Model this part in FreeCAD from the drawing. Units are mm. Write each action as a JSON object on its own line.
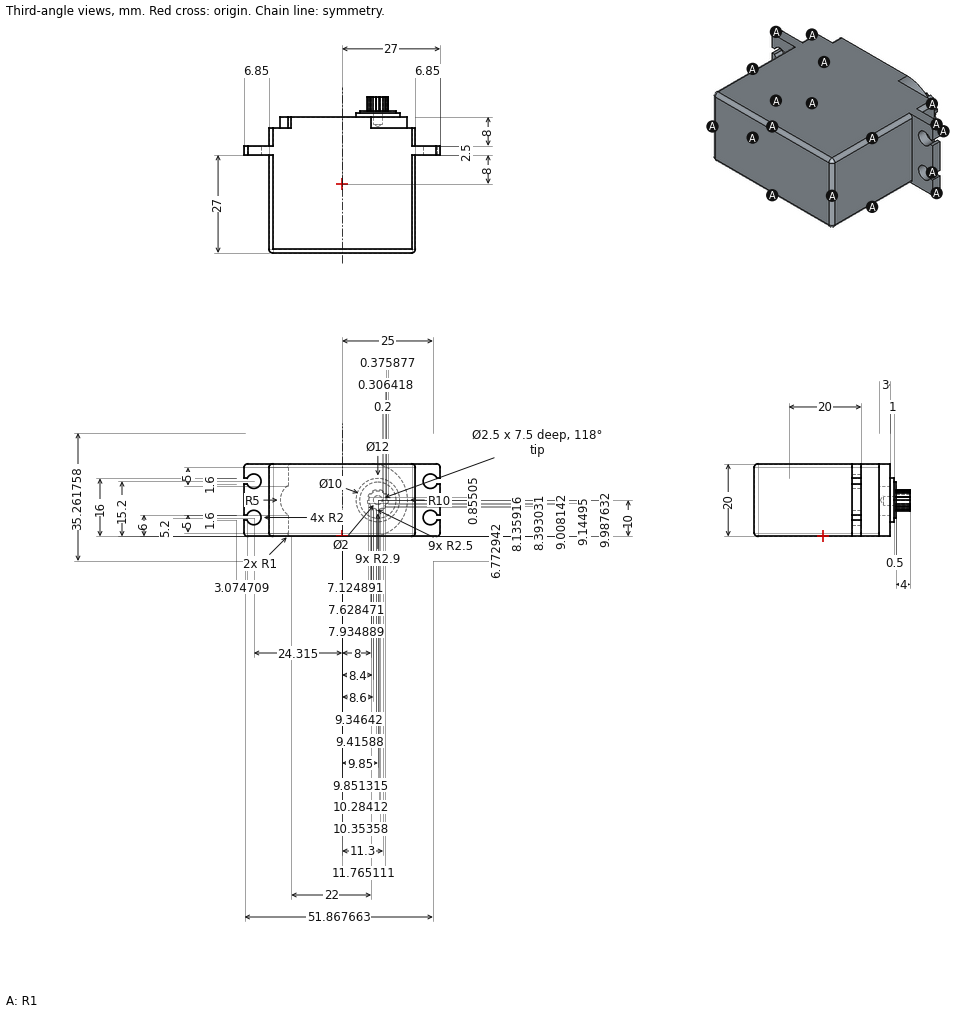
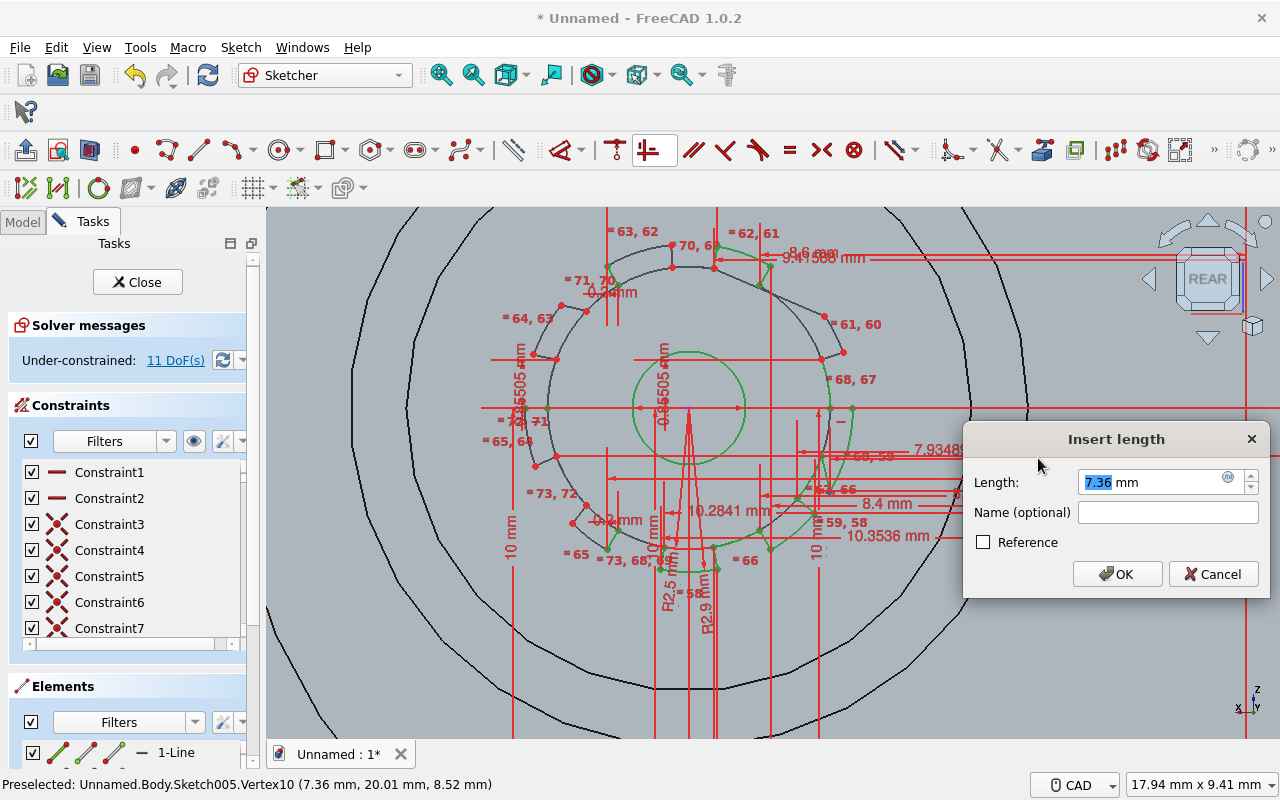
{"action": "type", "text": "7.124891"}
{"action": "key", "text": "Return"}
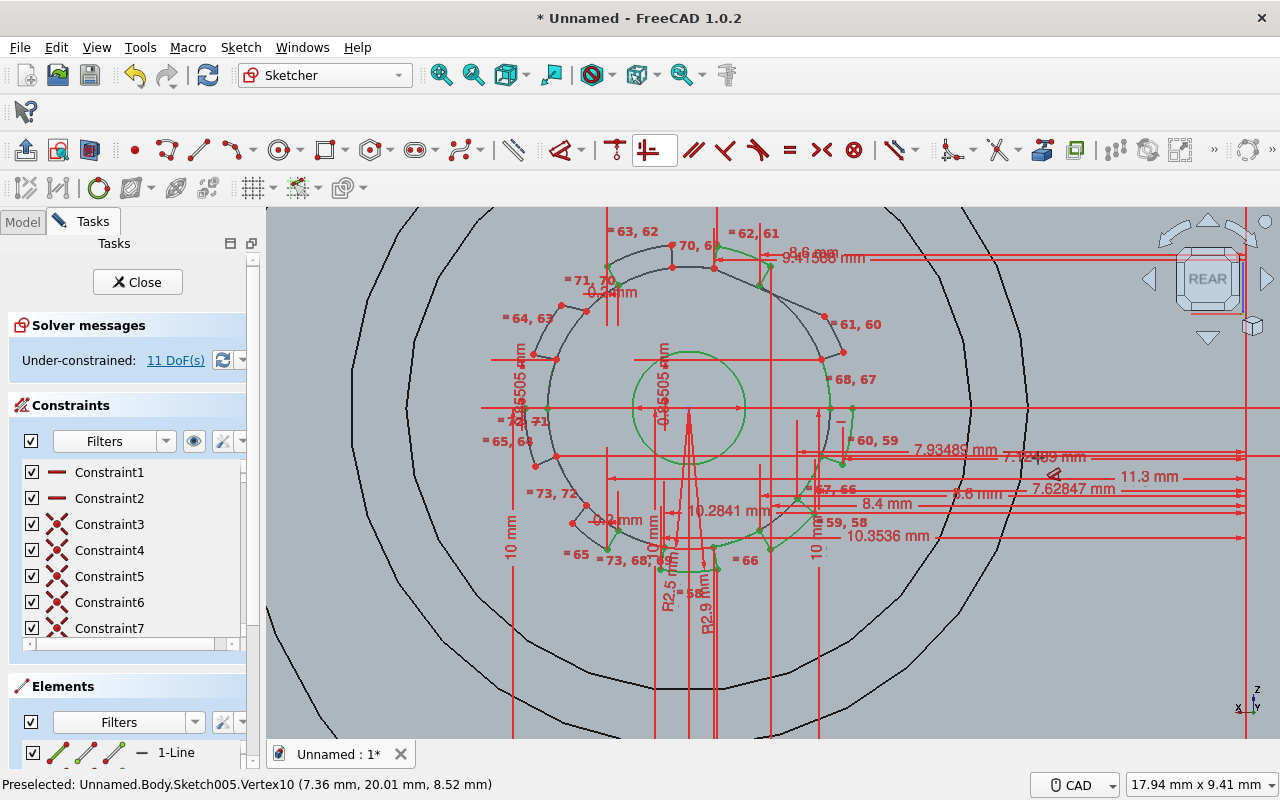
{"action": "left_click", "coordinate": [843, 353]}
{"action": "left_click", "coordinate": [979, 319]}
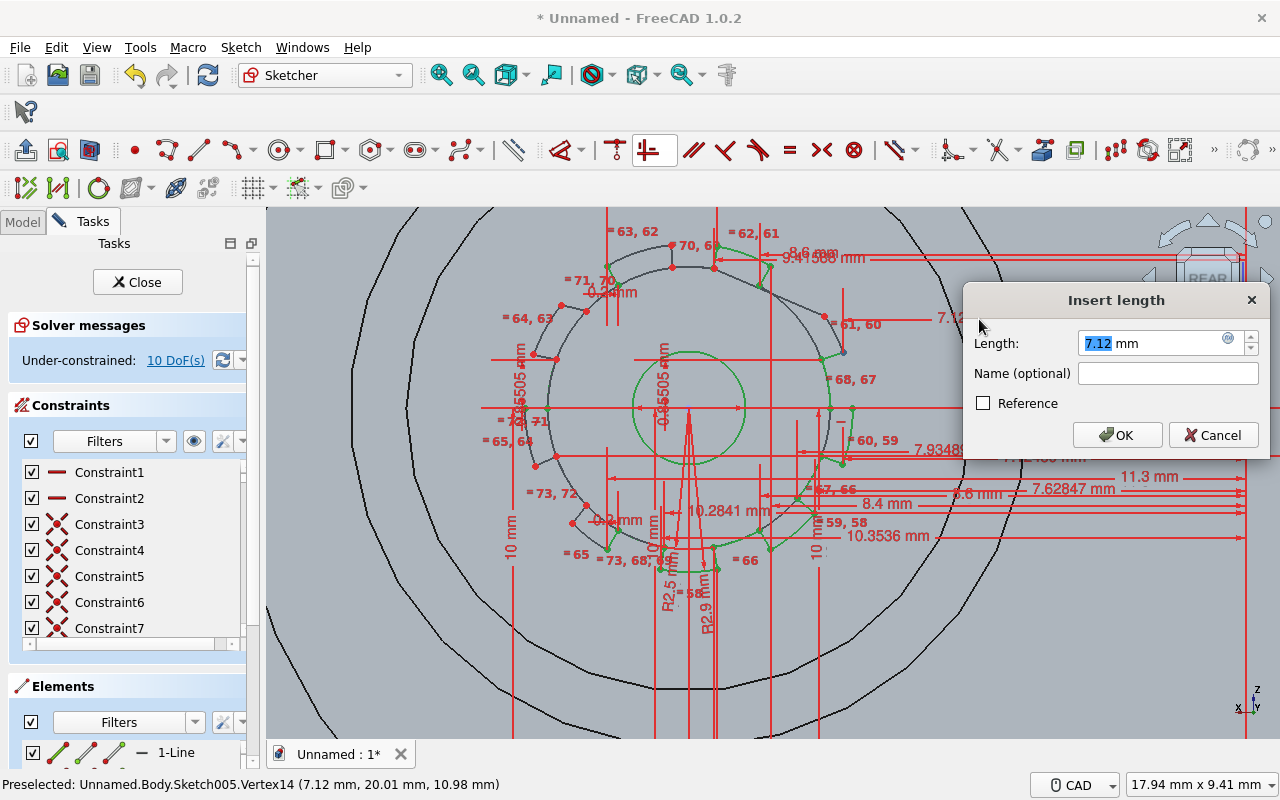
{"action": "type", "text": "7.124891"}
{"action": "key", "text": "Return"}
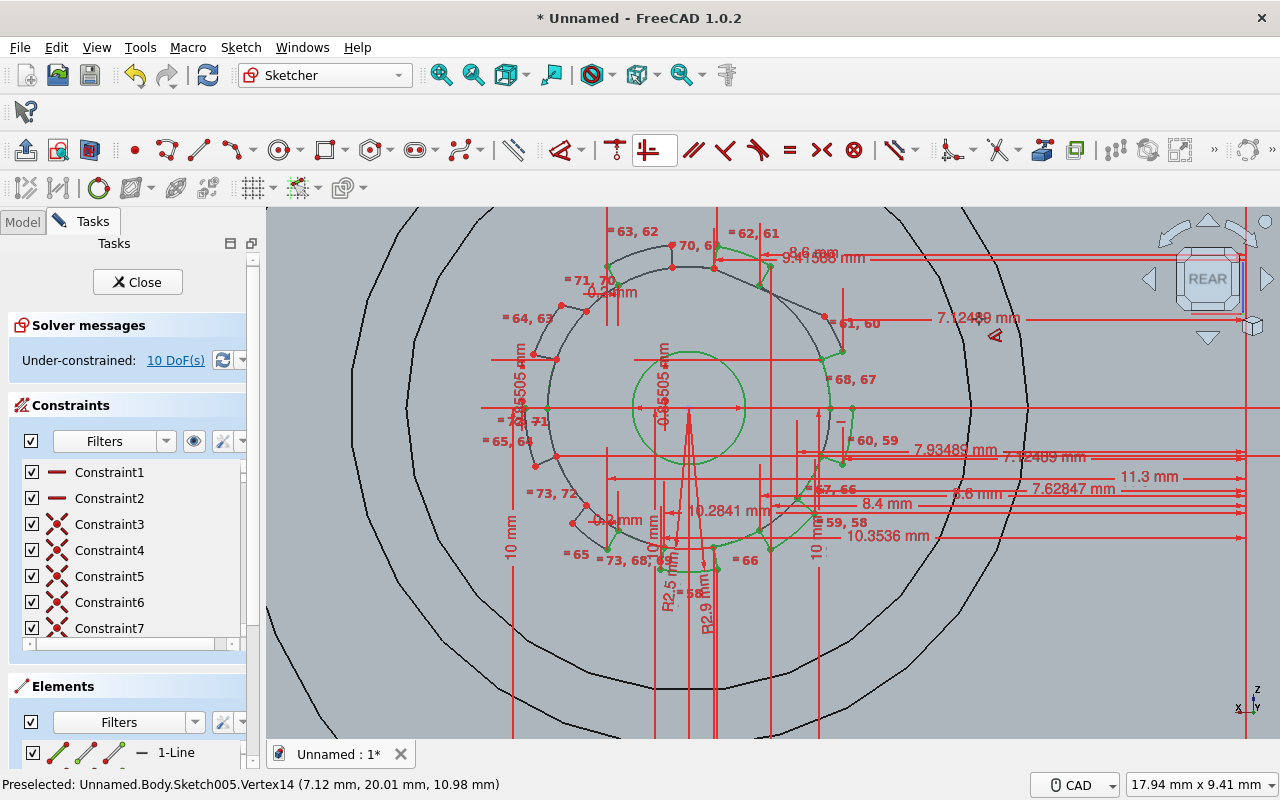
{"action": "left_click", "coordinate": [825, 316]}
{"action": "left_click", "coordinate": [970, 282]}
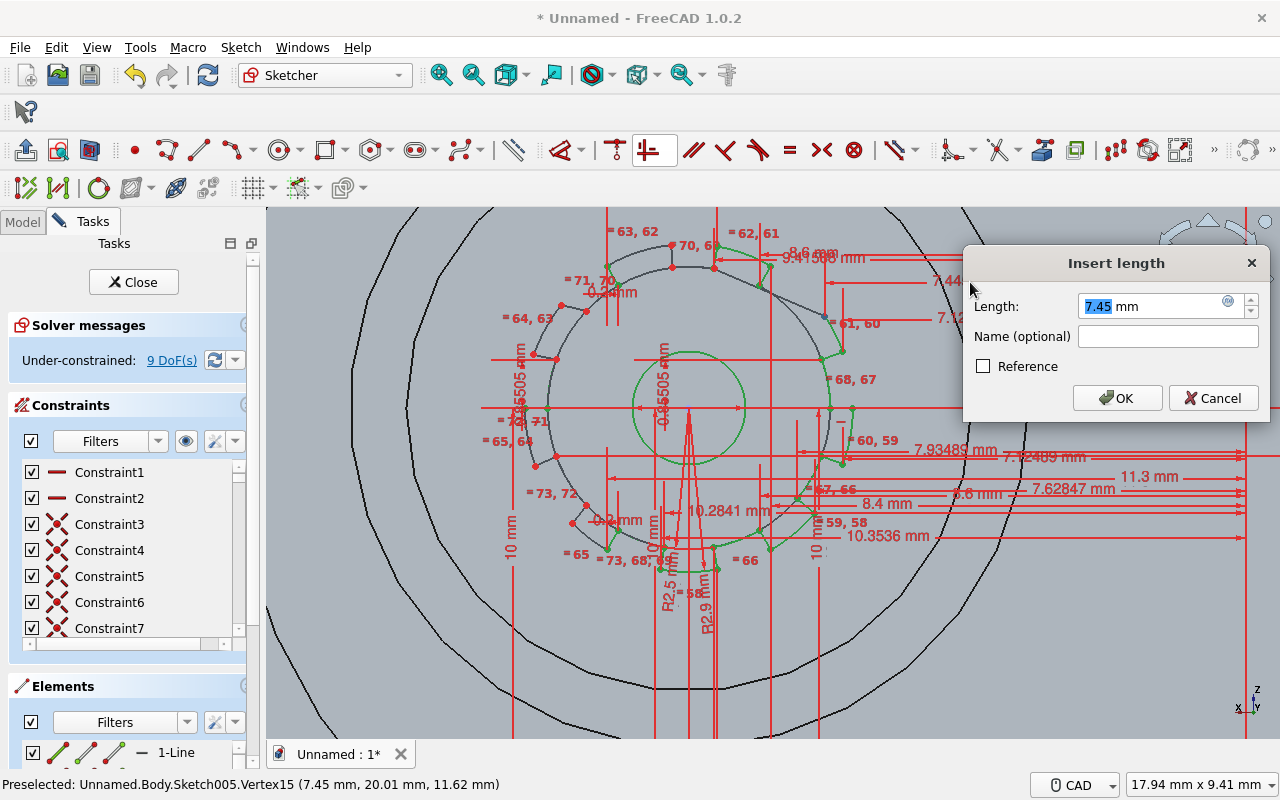
{"action": "type", "text": "7.628471"}
{"action": "key", "text": "Return"}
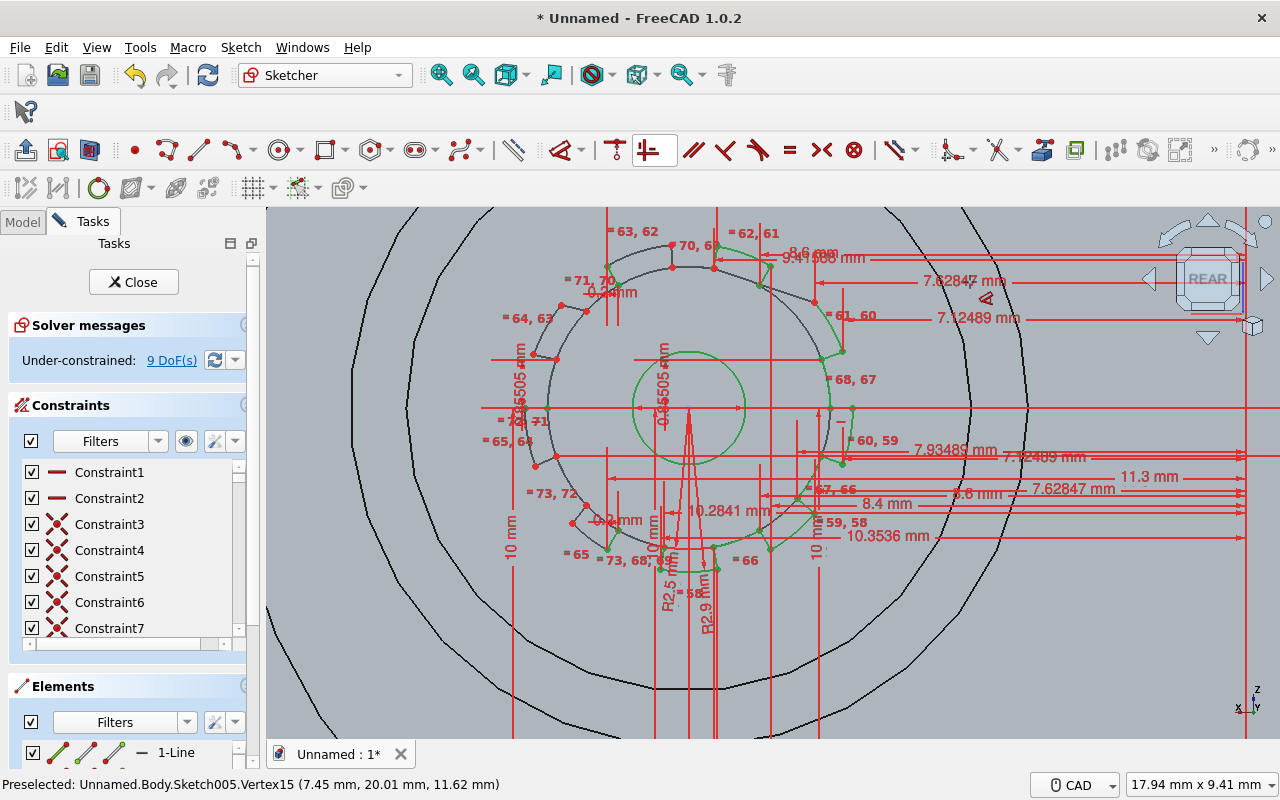
{"action": "scroll", "coordinate": [714, 269], "scroll_direction": "up", "scroll_amount": 10}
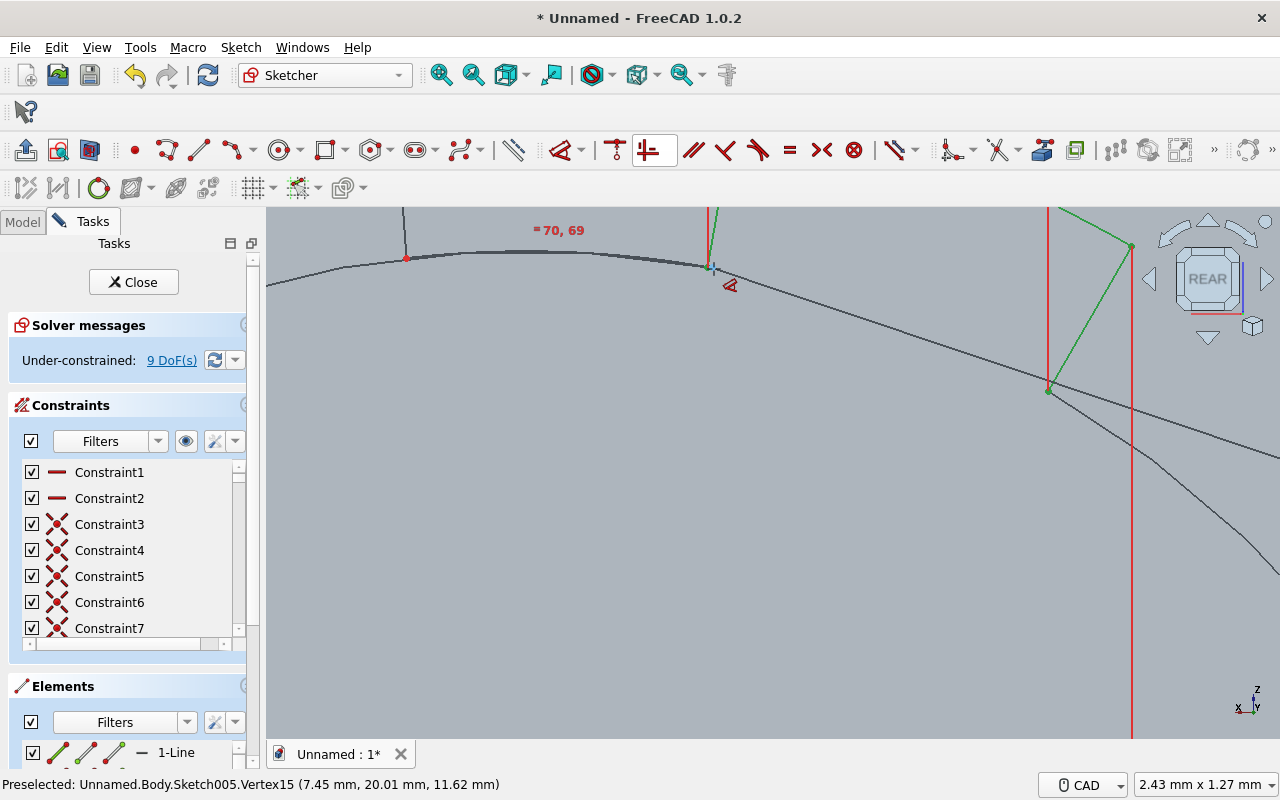
{"action": "left_click", "coordinate": [712, 268]}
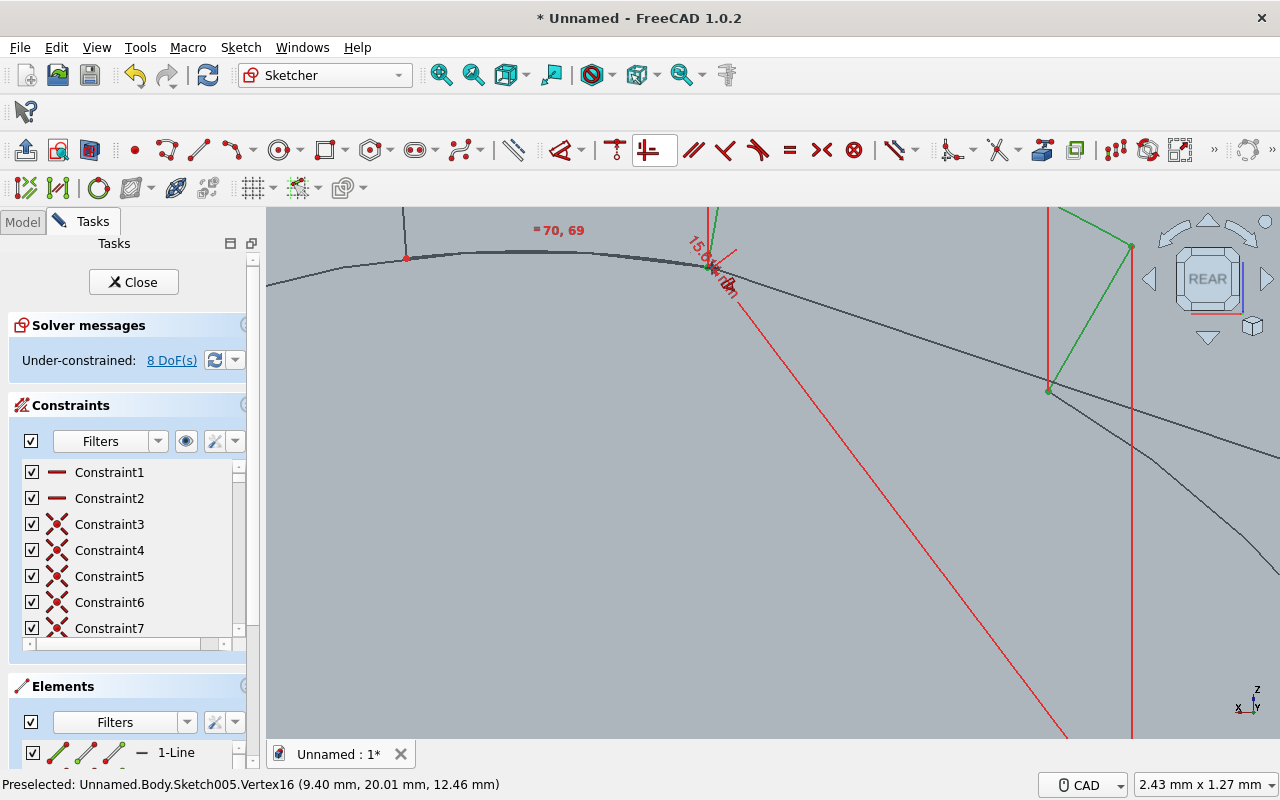
{"action": "key", "text": "Escape"}
{"action": "key", "text": "Escape"}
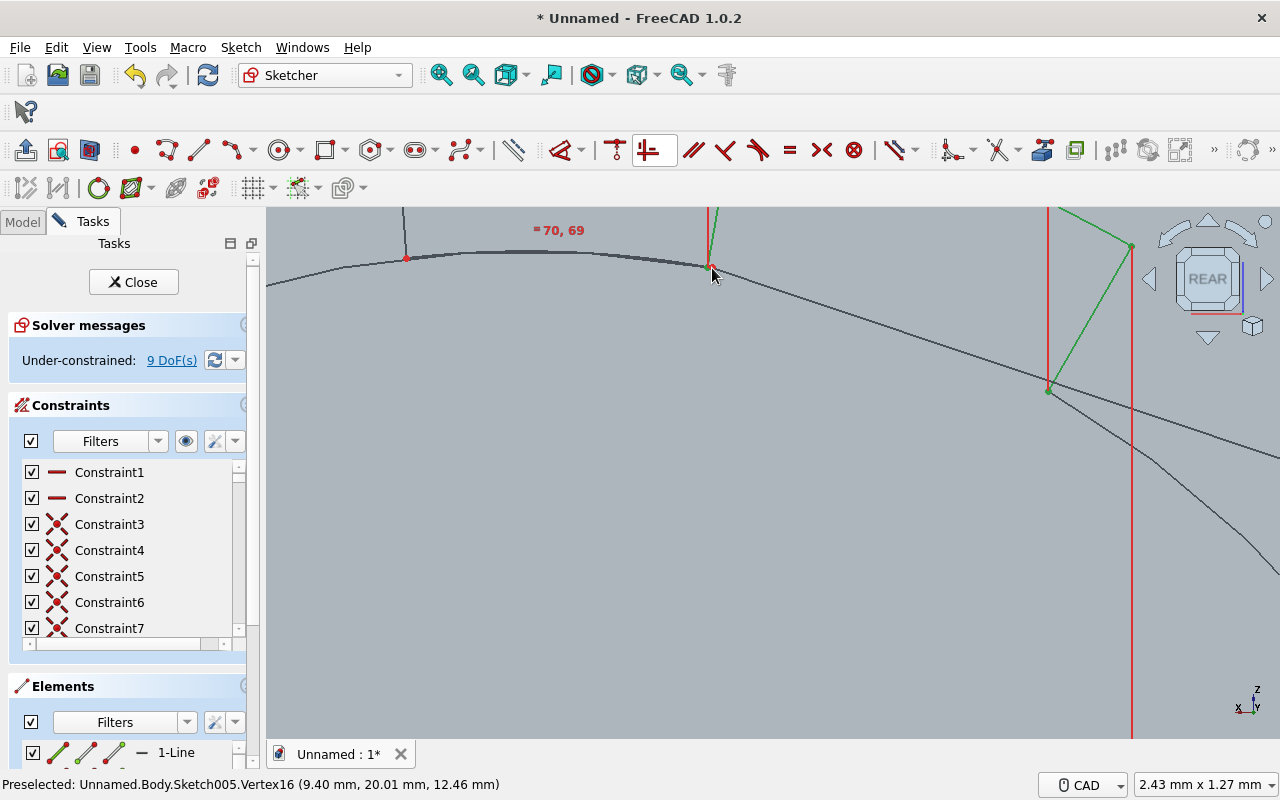
{"action": "left_click", "coordinate": [712, 268]}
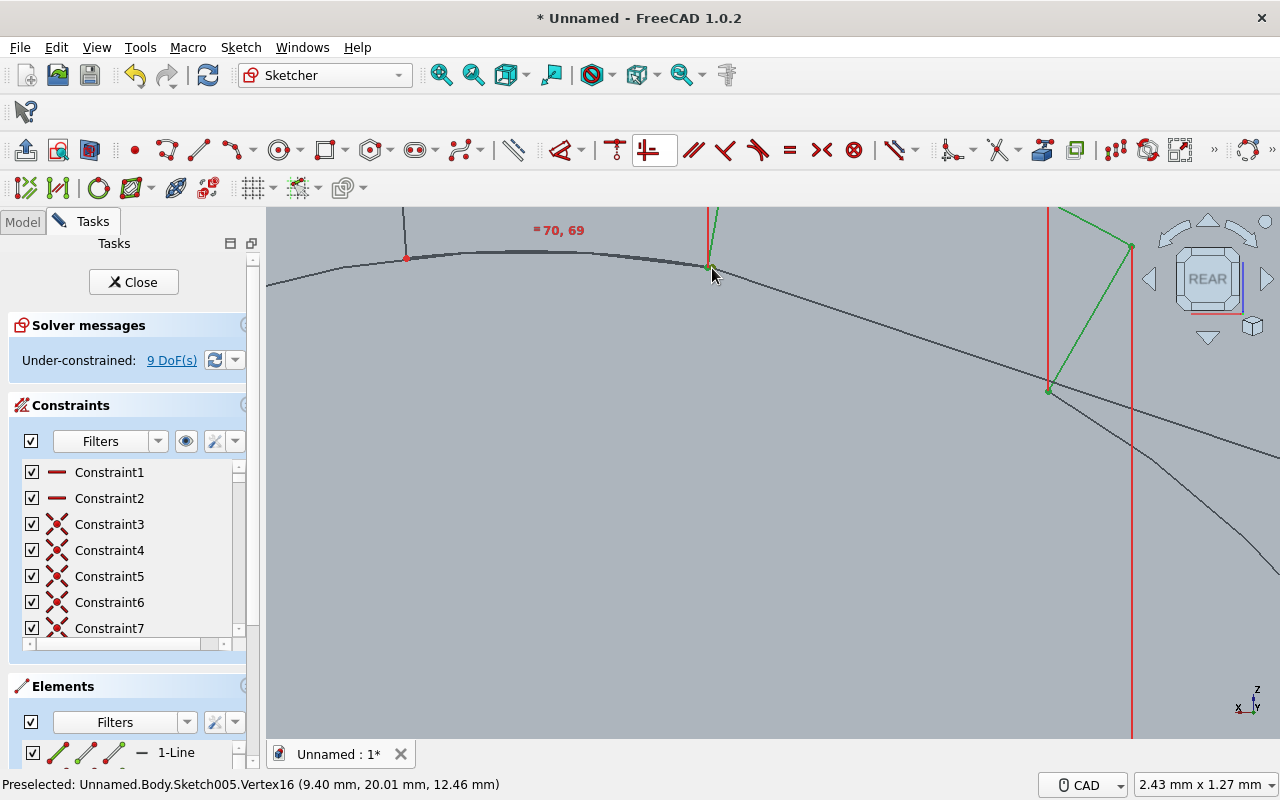
{"action": "left_click", "coordinate": [584, 150]}